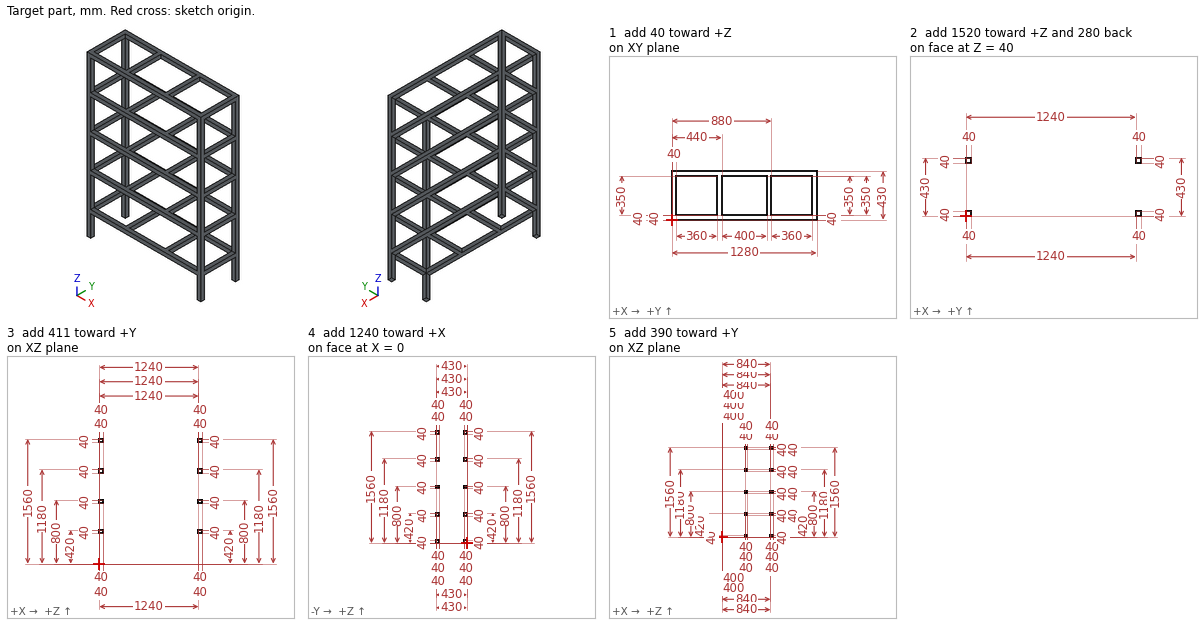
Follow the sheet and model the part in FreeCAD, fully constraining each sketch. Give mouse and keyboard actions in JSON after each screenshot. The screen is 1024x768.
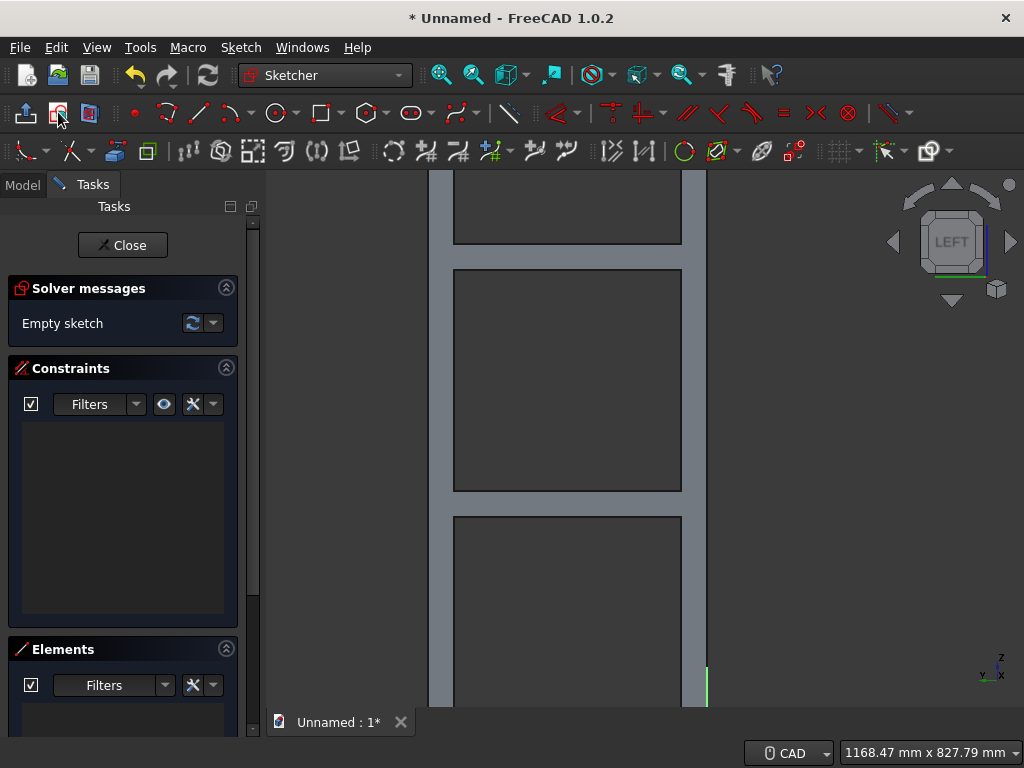
{"action": "scroll", "coordinate": [582, 544], "scroll_direction": "down", "scroll_amount": 5}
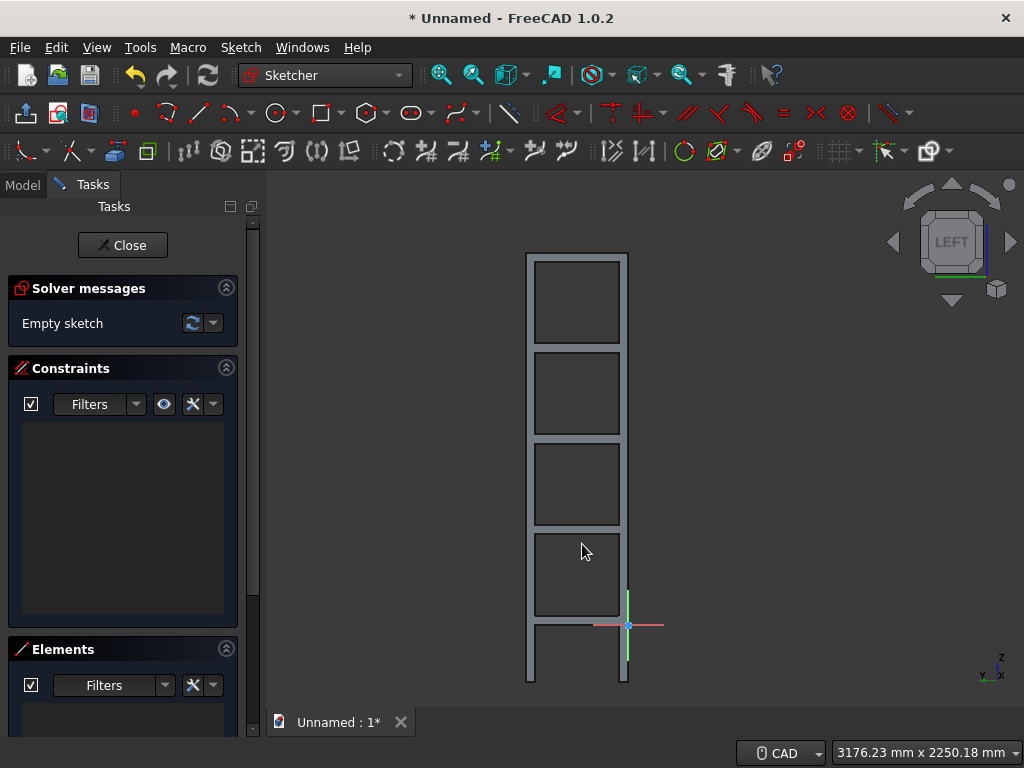
{"action": "left_click", "coordinate": [322, 114]}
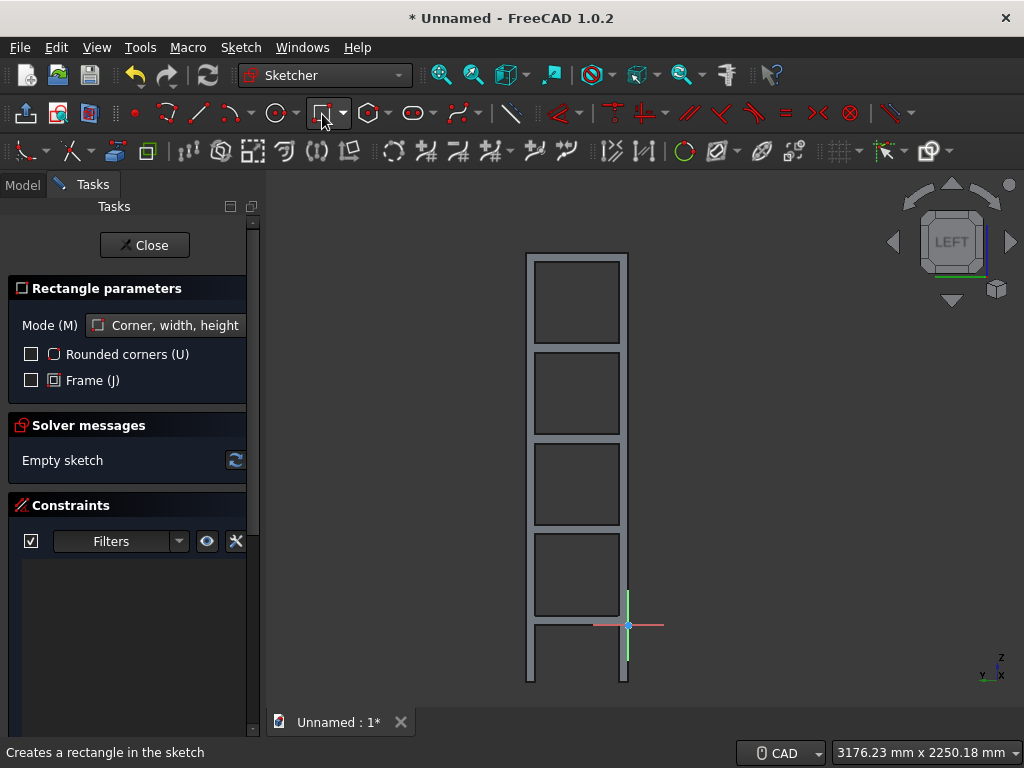
{"action": "scroll", "coordinate": [526, 616], "scroll_direction": "up", "scroll_amount": 3}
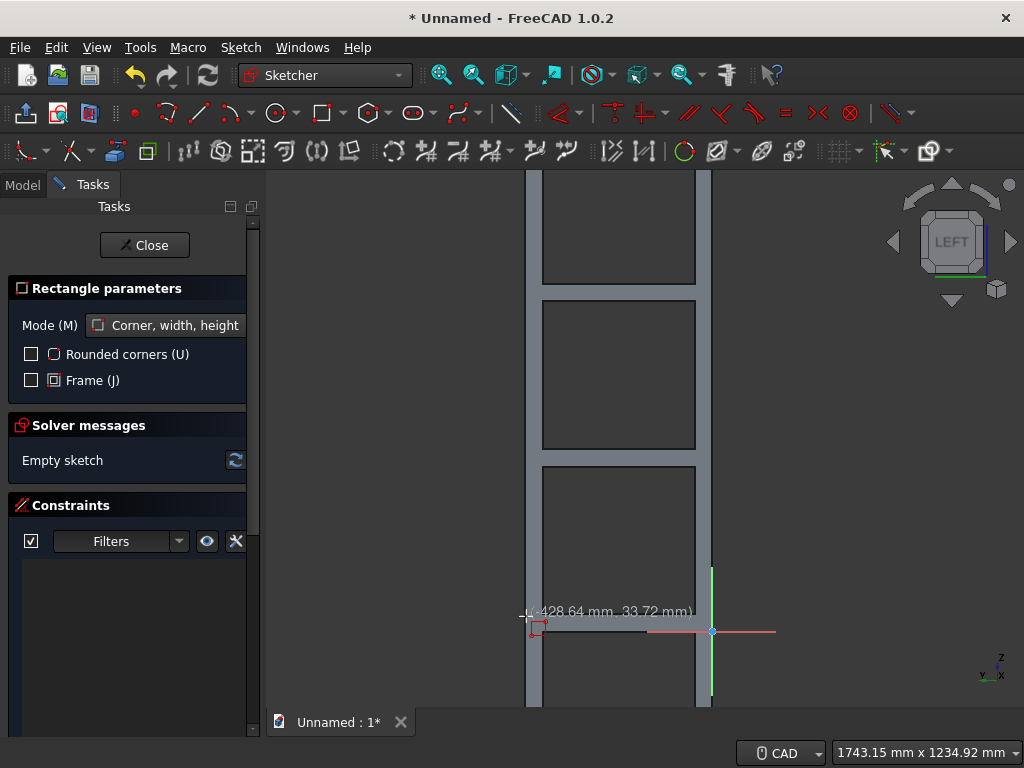
{"action": "left_click", "coordinate": [525, 614]}
{"action": "left_click", "coordinate": [543, 632]}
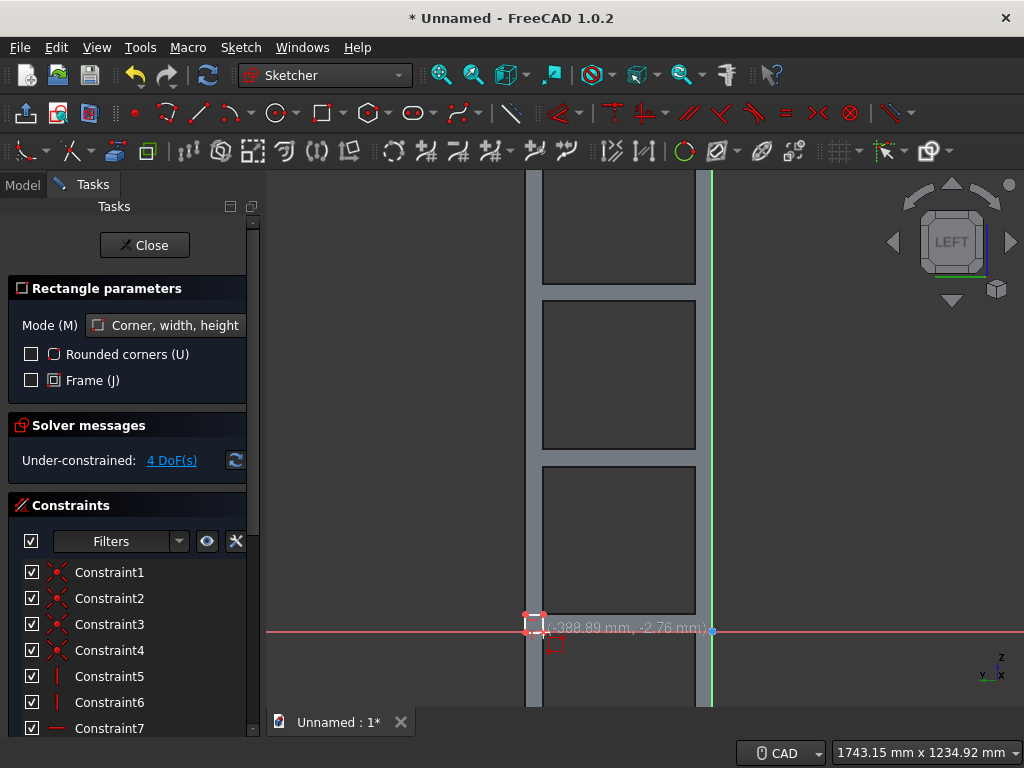
{"action": "left_click", "coordinate": [712, 632]}
{"action": "mouse_move", "coordinate": [695, 614]}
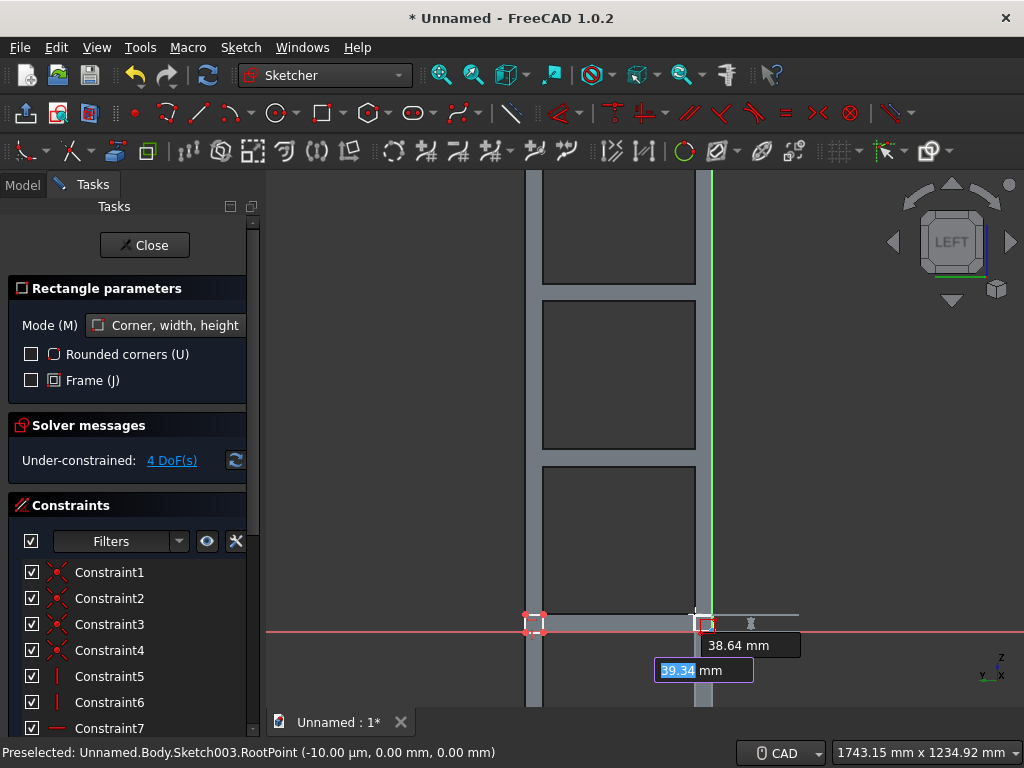
{"action": "type", "text": "40"}
{"action": "key", "text": "Tab"}
{"action": "type", "text": "40"}
{"action": "key", "text": "Return"}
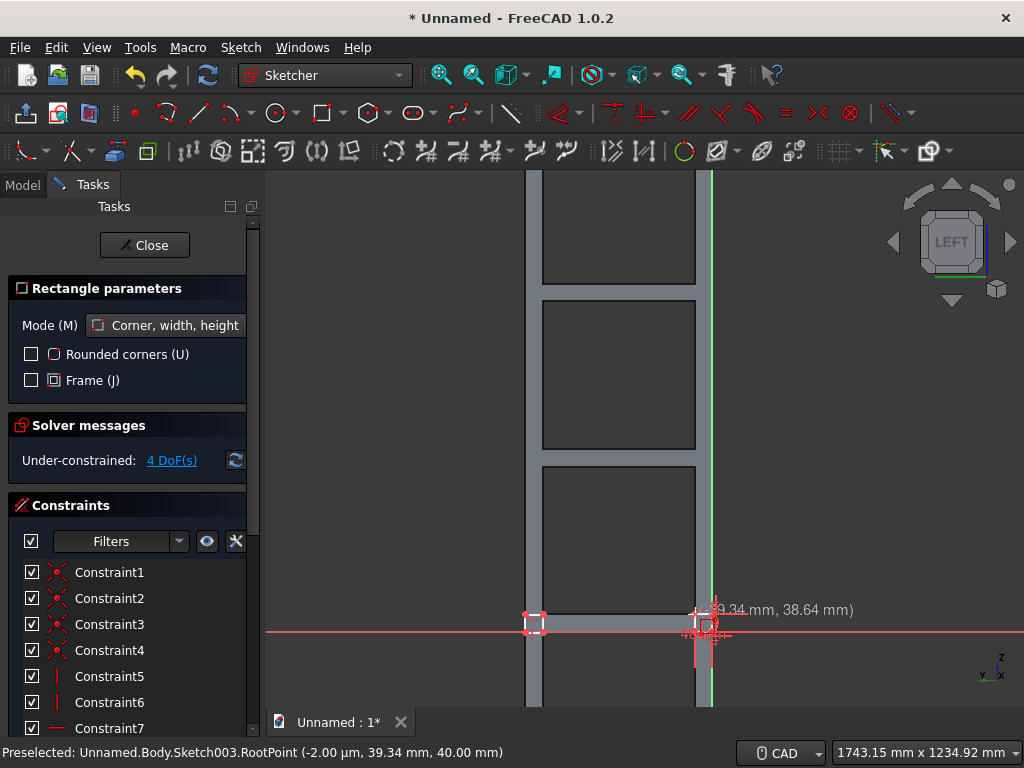
{"action": "left_click", "coordinate": [695, 449]}
{"action": "left_click", "coordinate": [712, 467]}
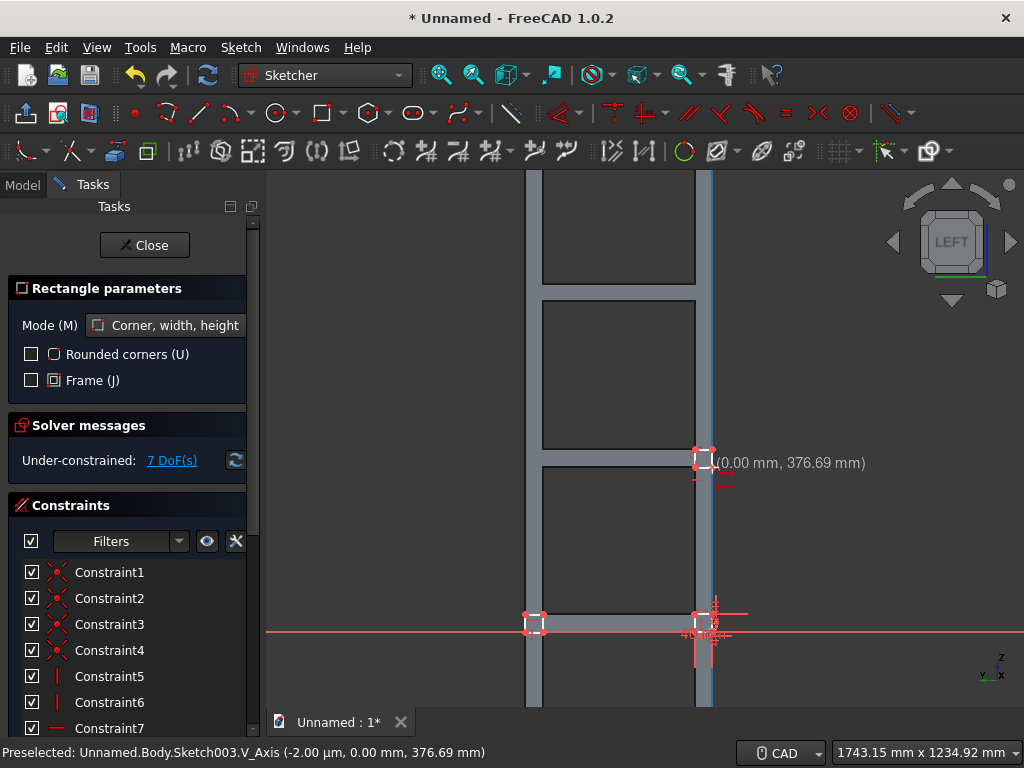
{"action": "left_click", "coordinate": [525, 449]}
{"action": "mouse_move", "coordinate": [543, 467]}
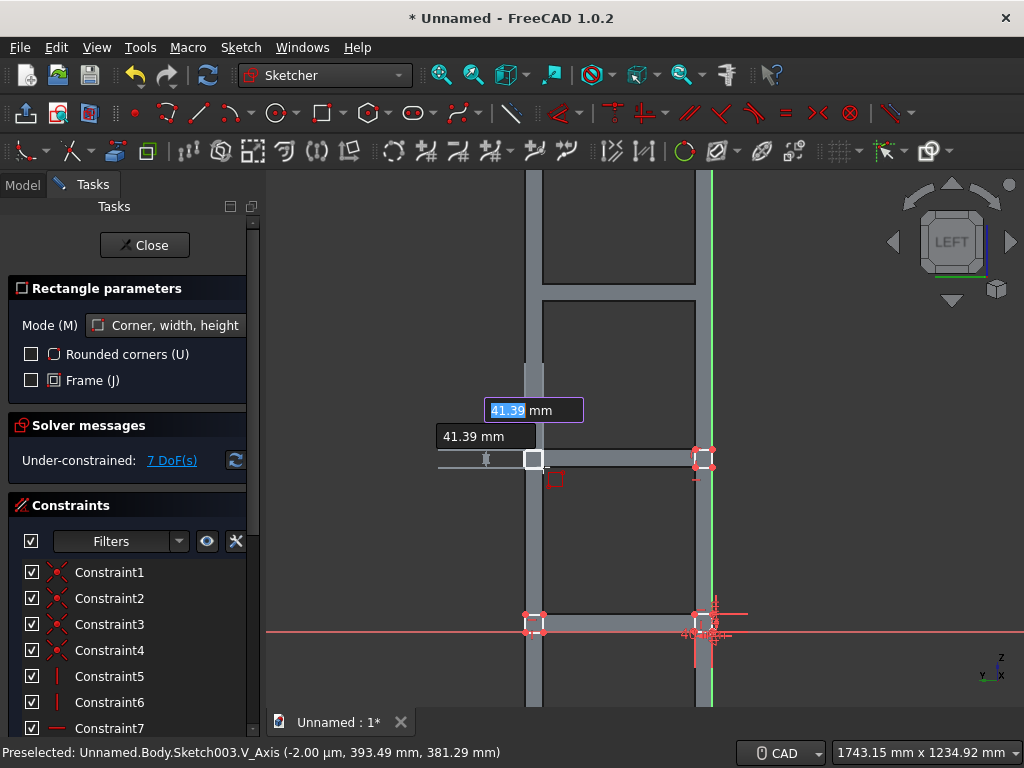
{"action": "type", "text": "40"}
{"action": "key", "text": "Tab"}
{"action": "type", "text": "40"}
{"action": "key", "text": "Return"}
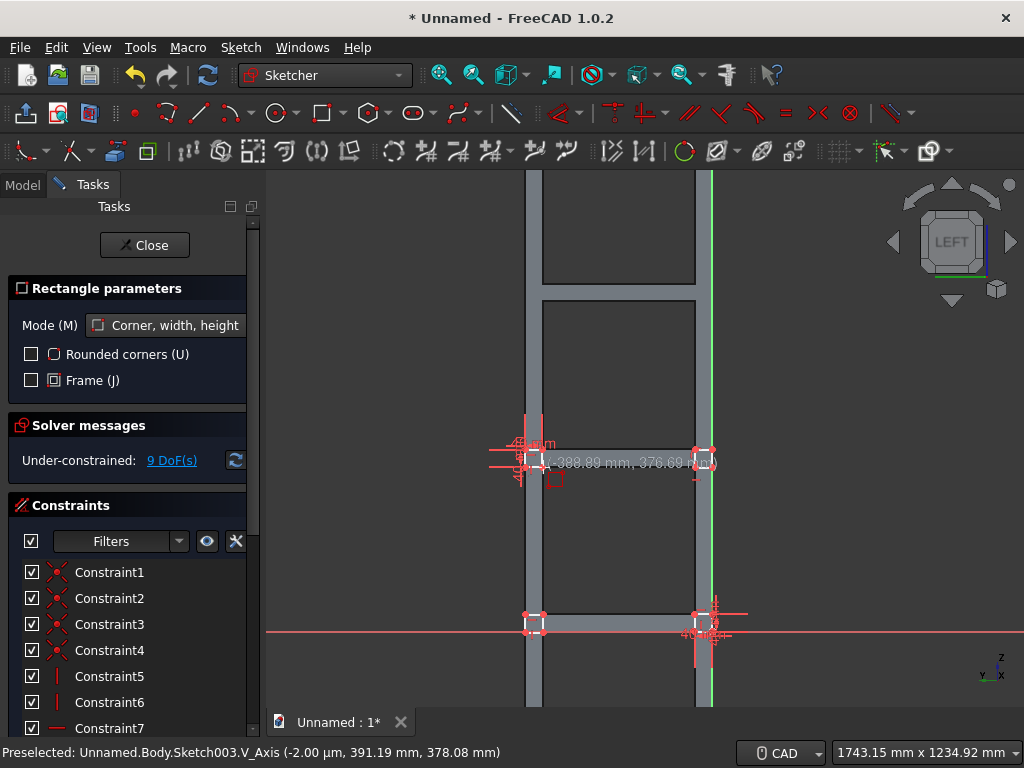
{"action": "left_click", "coordinate": [525, 284]}
{"action": "mouse_move", "coordinate": [543, 301]}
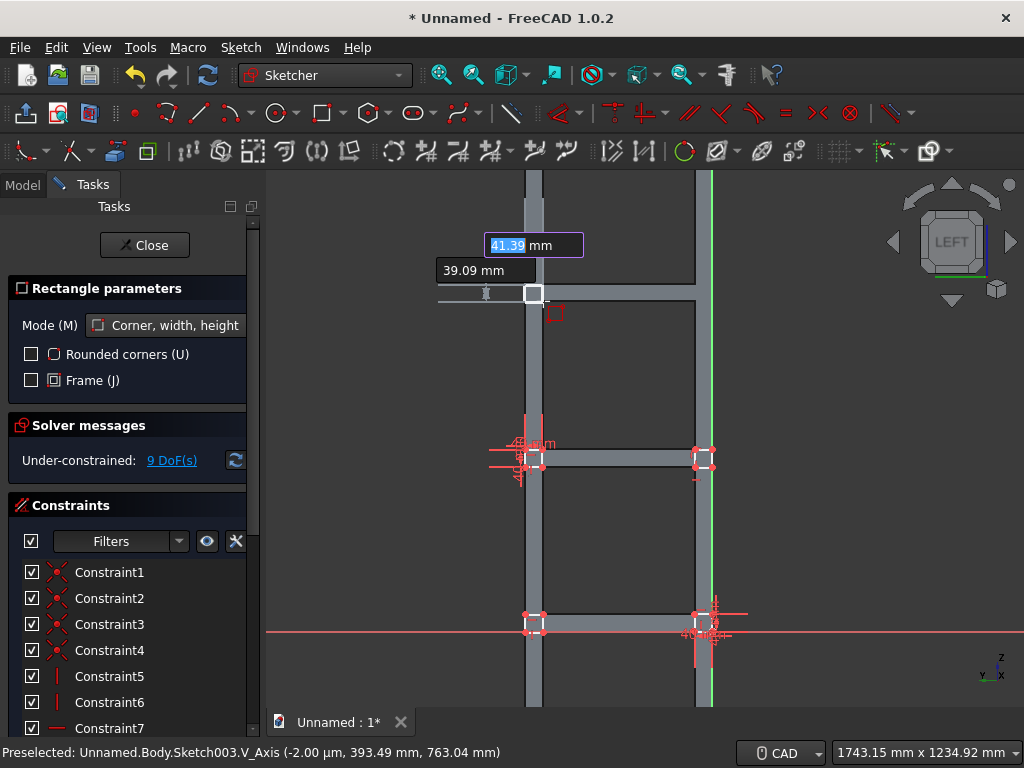
{"action": "type", "text": "40"}
{"action": "key", "text": "Tab"}
{"action": "type", "text": "40"}
{"action": "key", "text": "Return"}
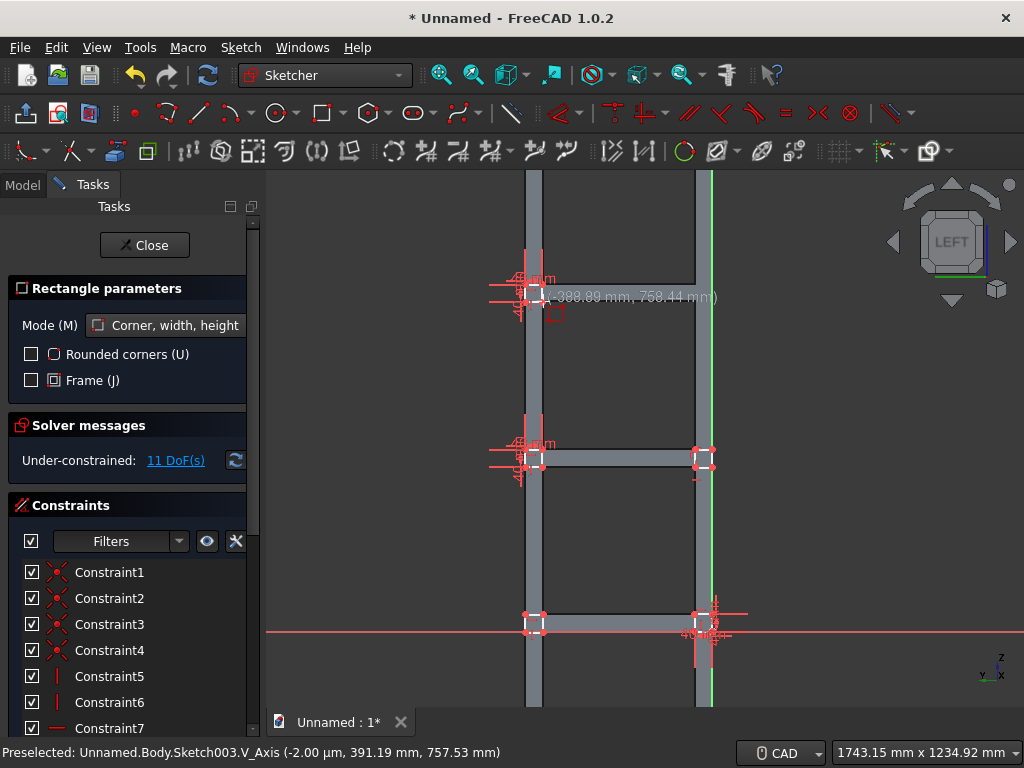
{"action": "left_click", "coordinate": [695, 284]}
{"action": "left_click", "coordinate": [712, 301]}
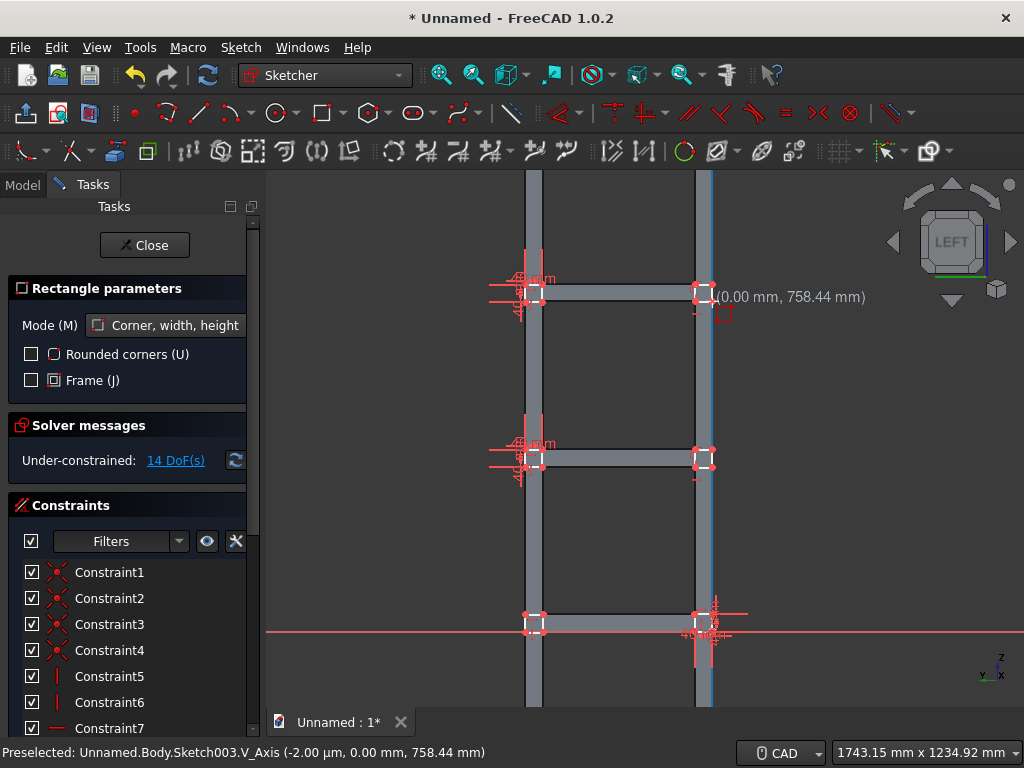
{"action": "scroll", "coordinate": [525, 616], "scroll_direction": "down", "scroll_amount": 3}